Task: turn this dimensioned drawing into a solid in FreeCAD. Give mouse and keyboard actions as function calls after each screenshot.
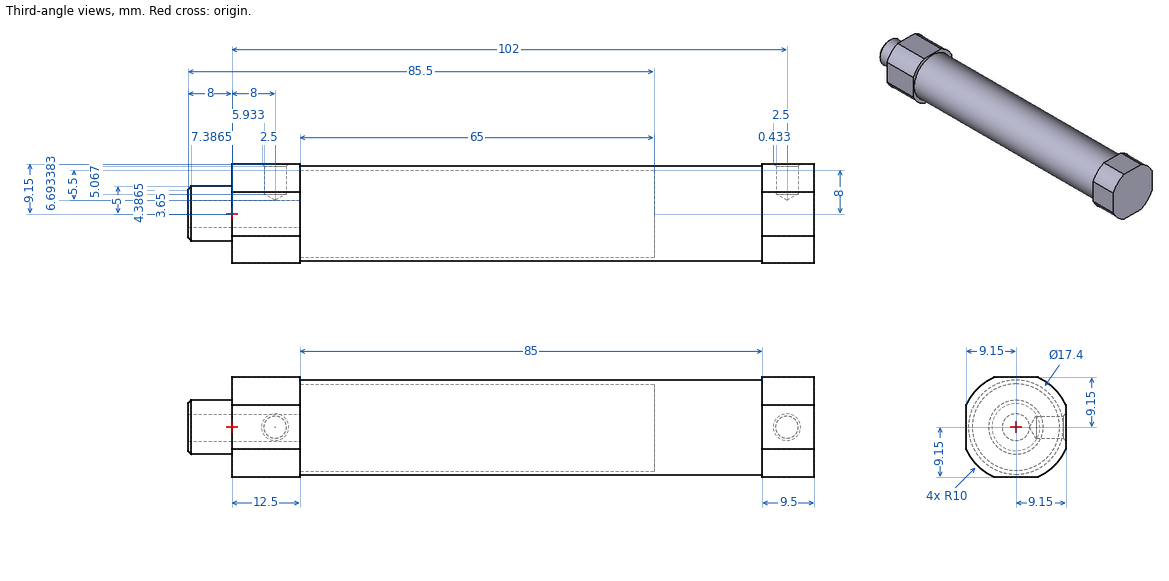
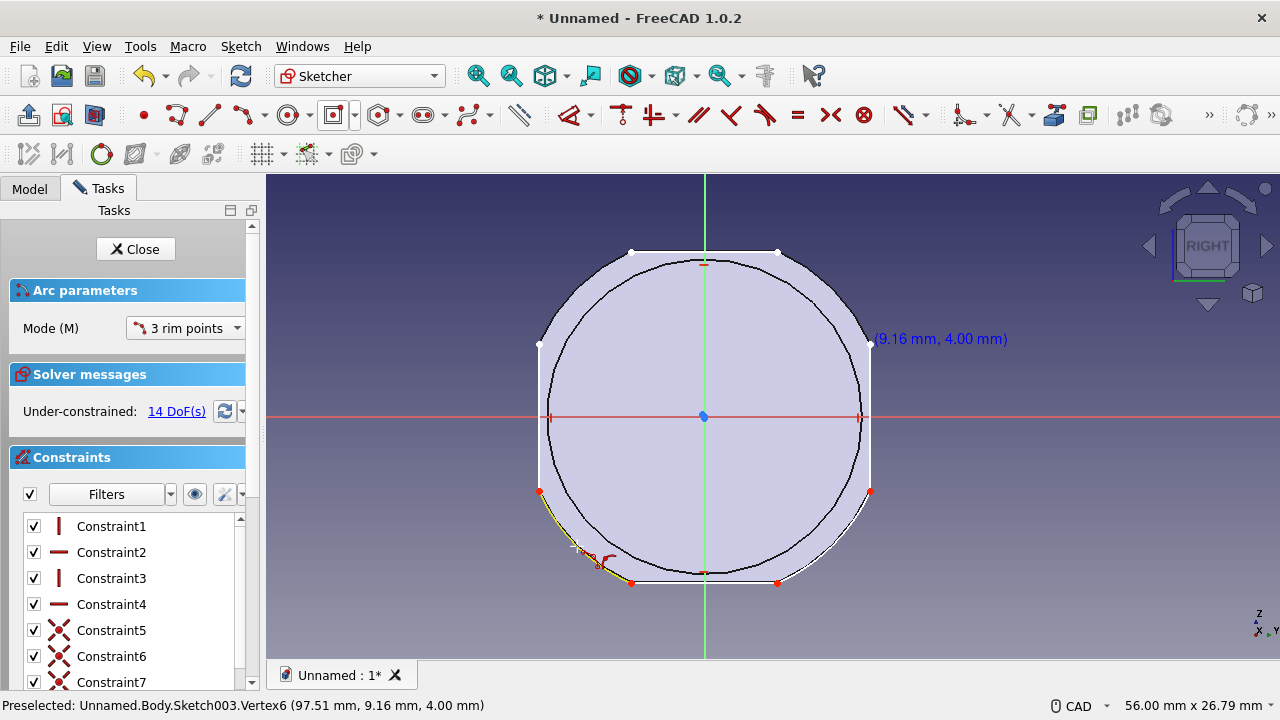
click(777, 252)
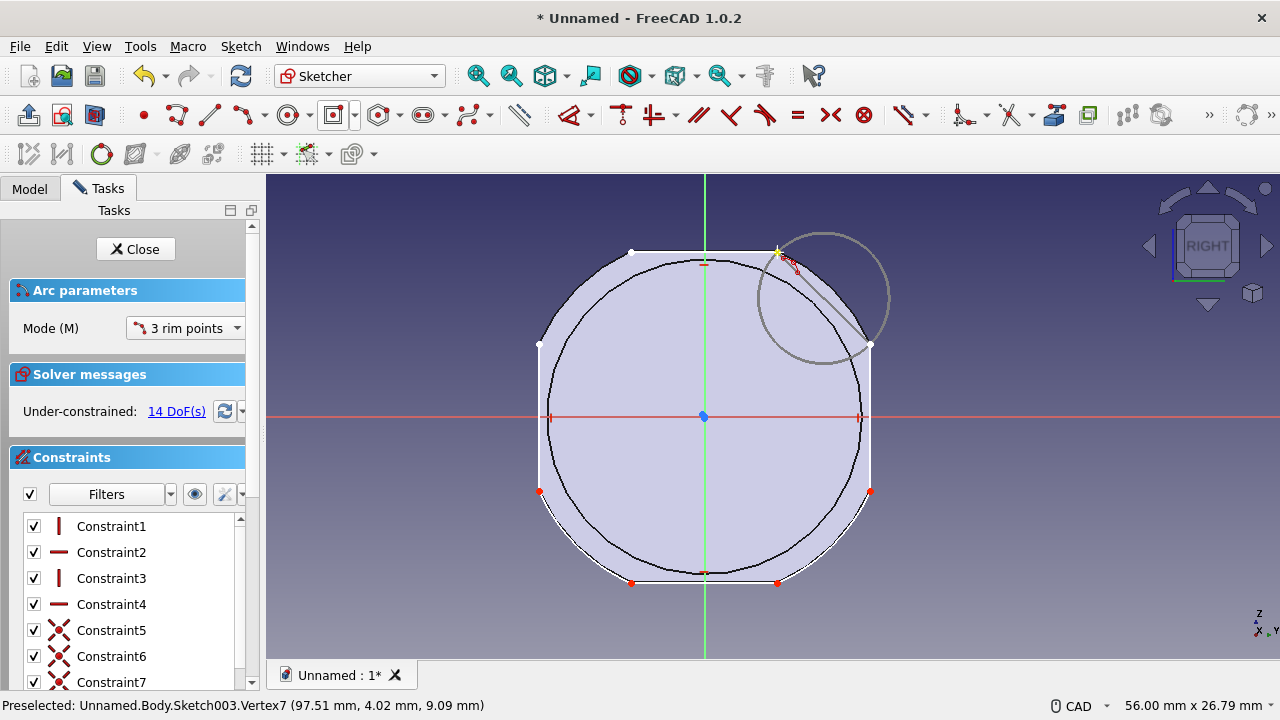
scroll(833, 289, up, 2)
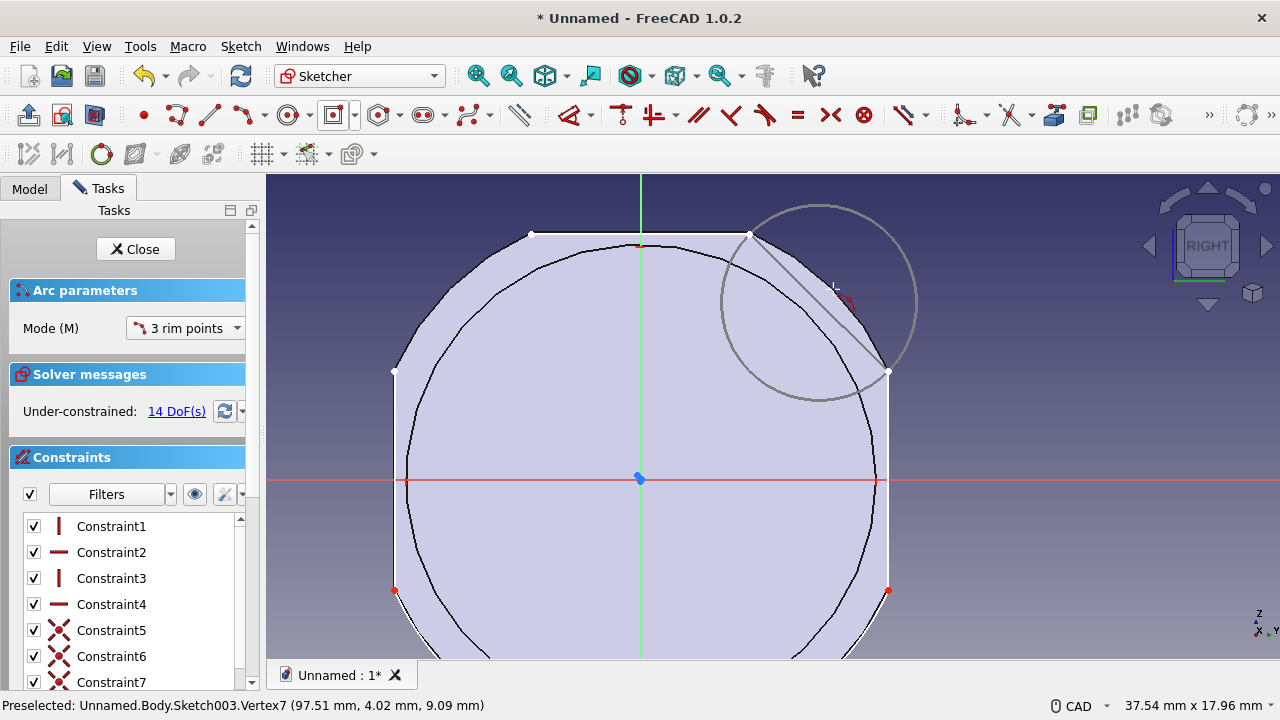
click(832, 289)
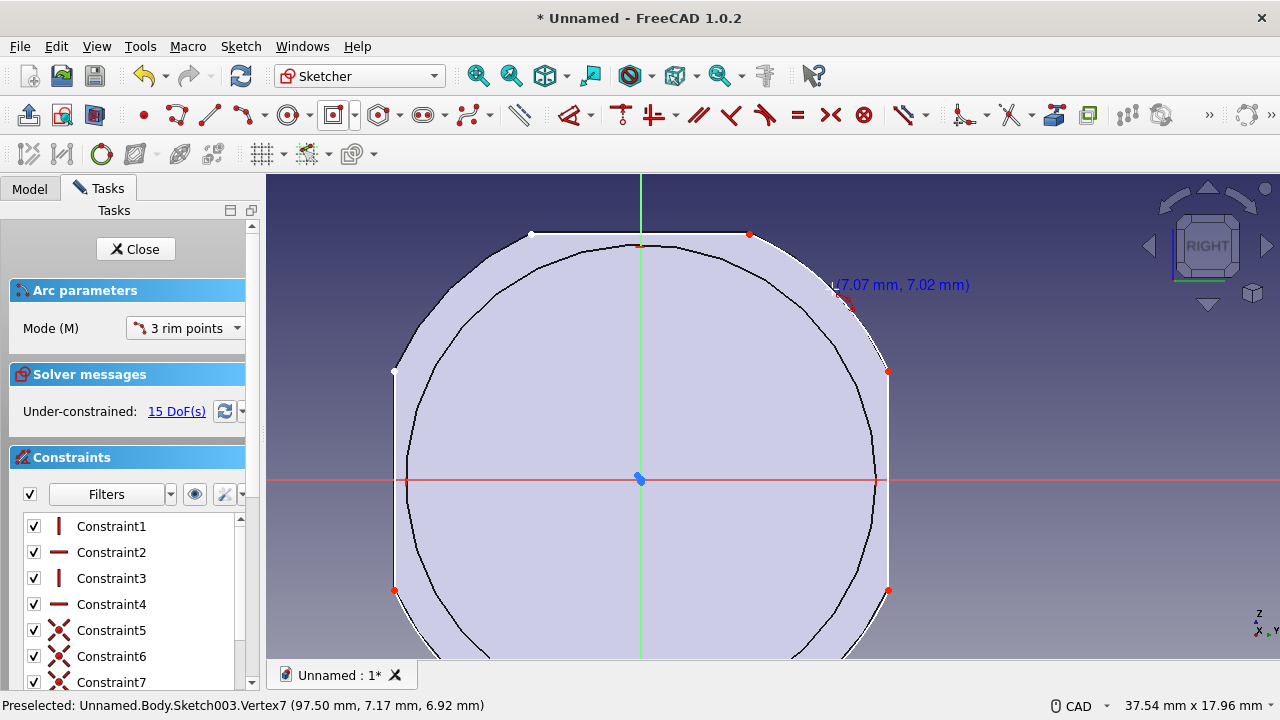
click(532, 234)
click(395, 371)
click(450, 289)
key(Escape)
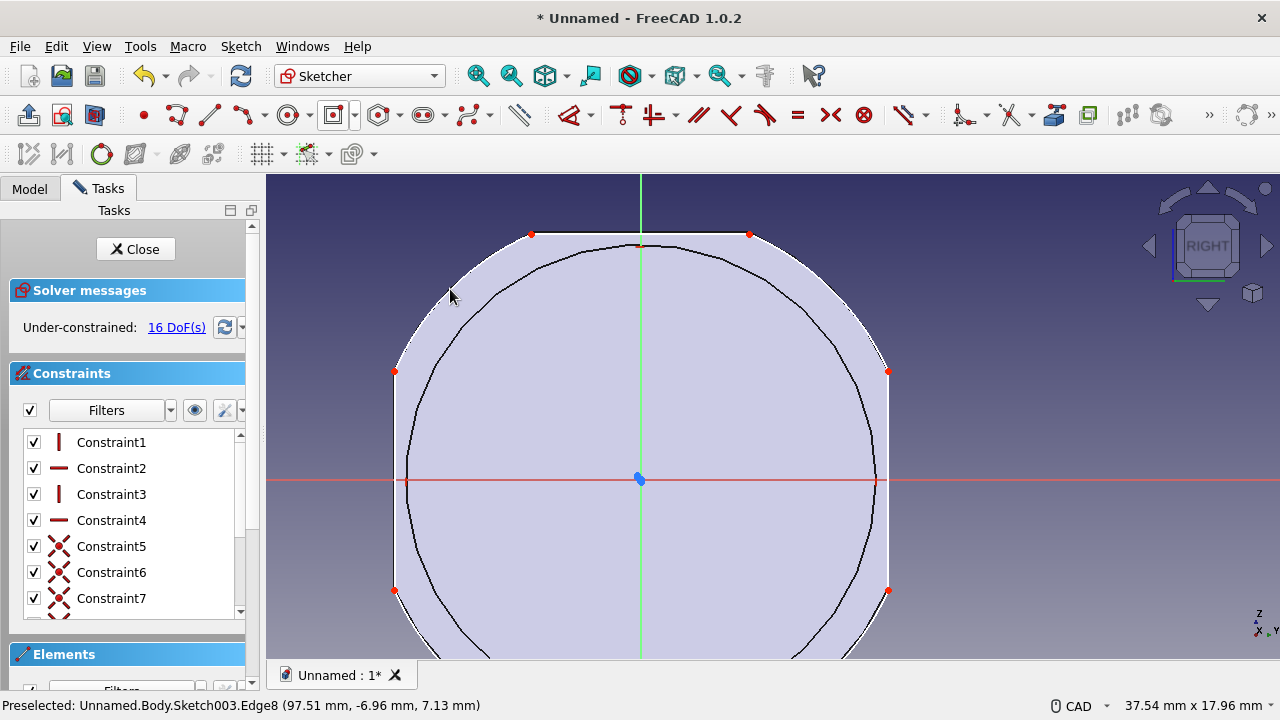
click(413, 626)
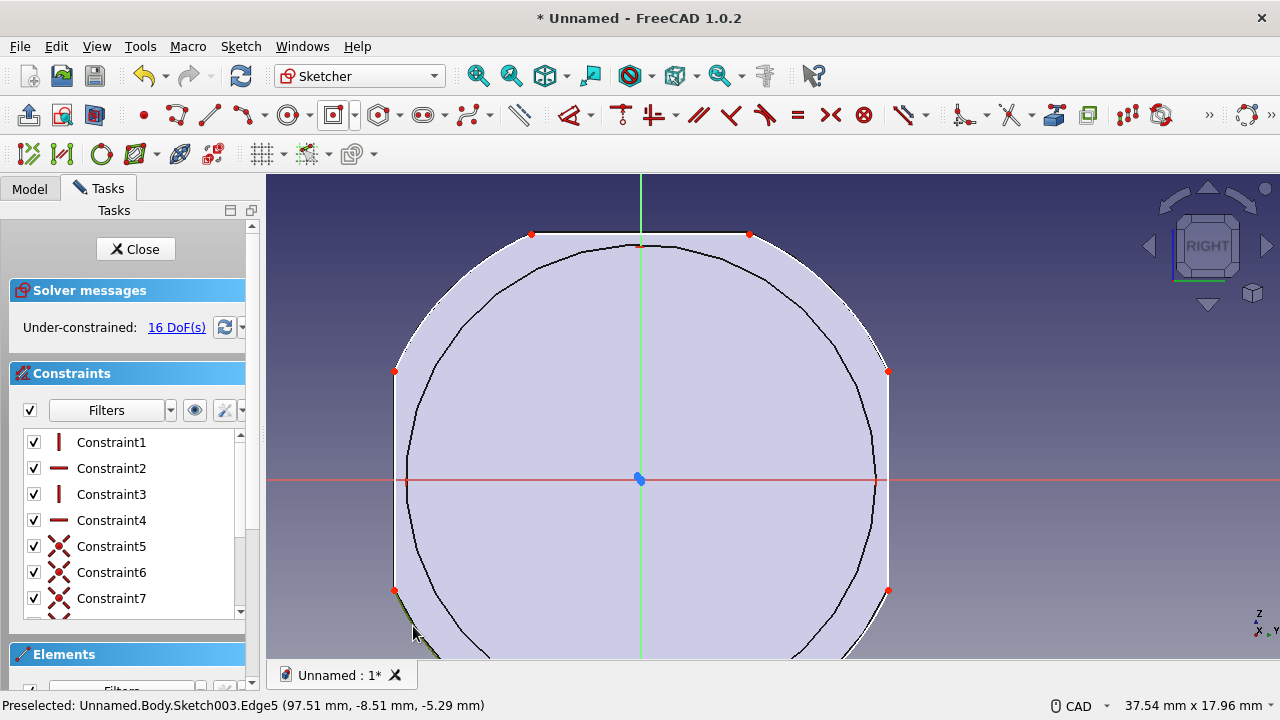
click(869, 626)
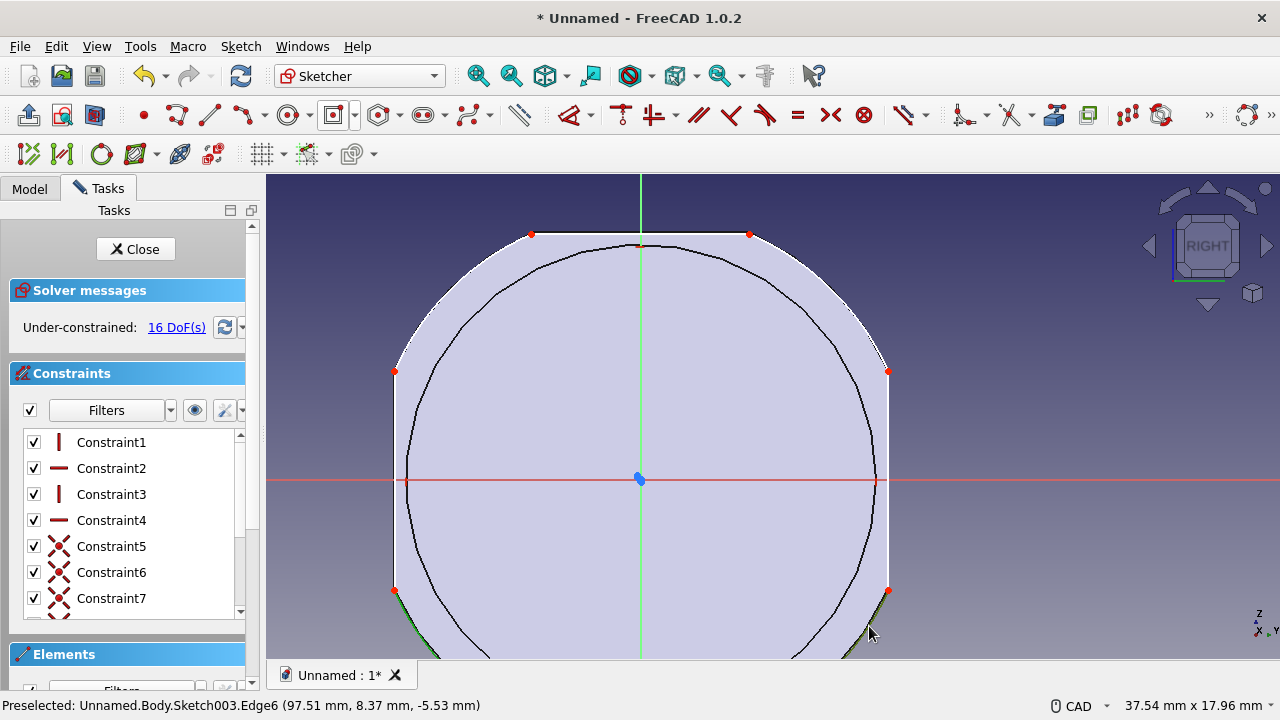
click(621, 116)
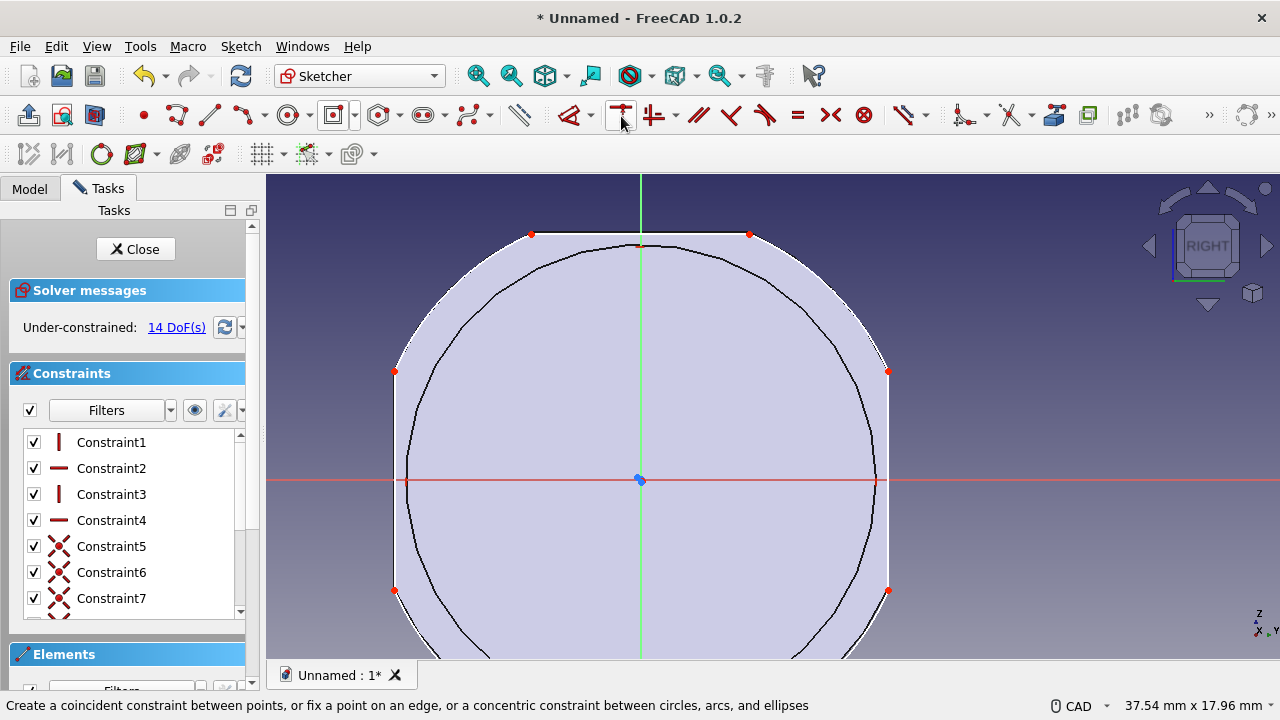
click(413, 626)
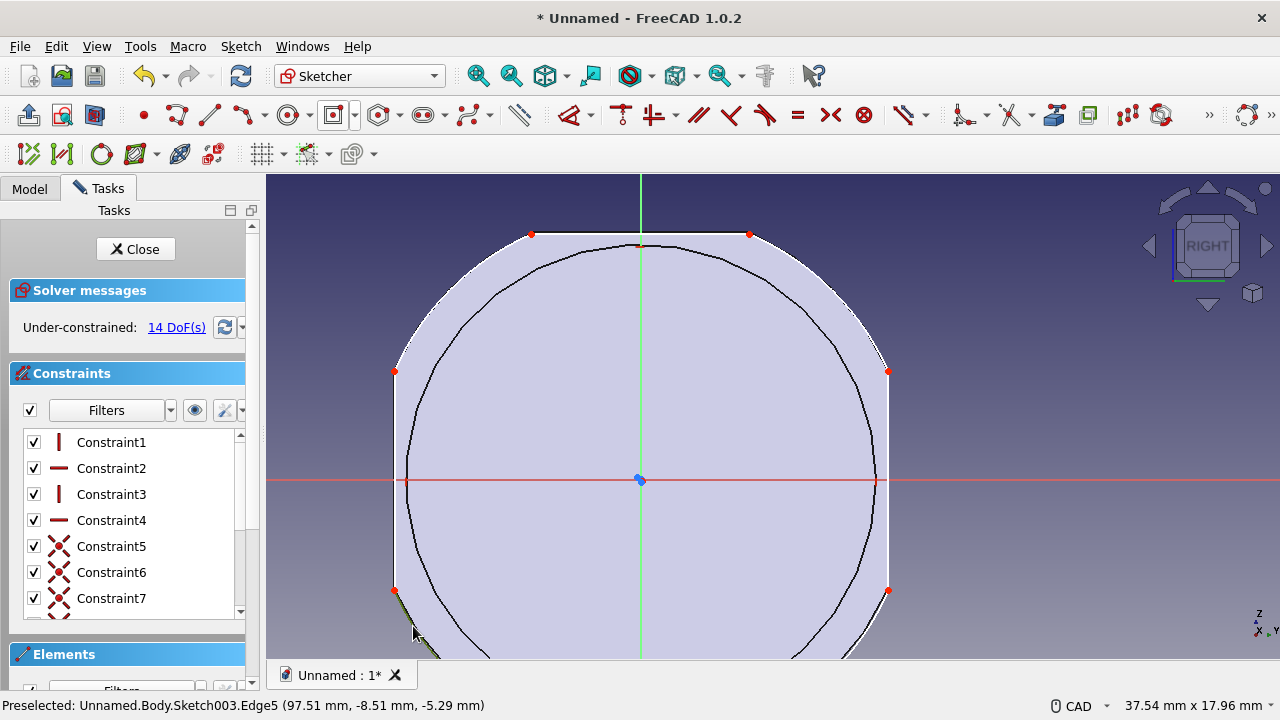
click(858, 320)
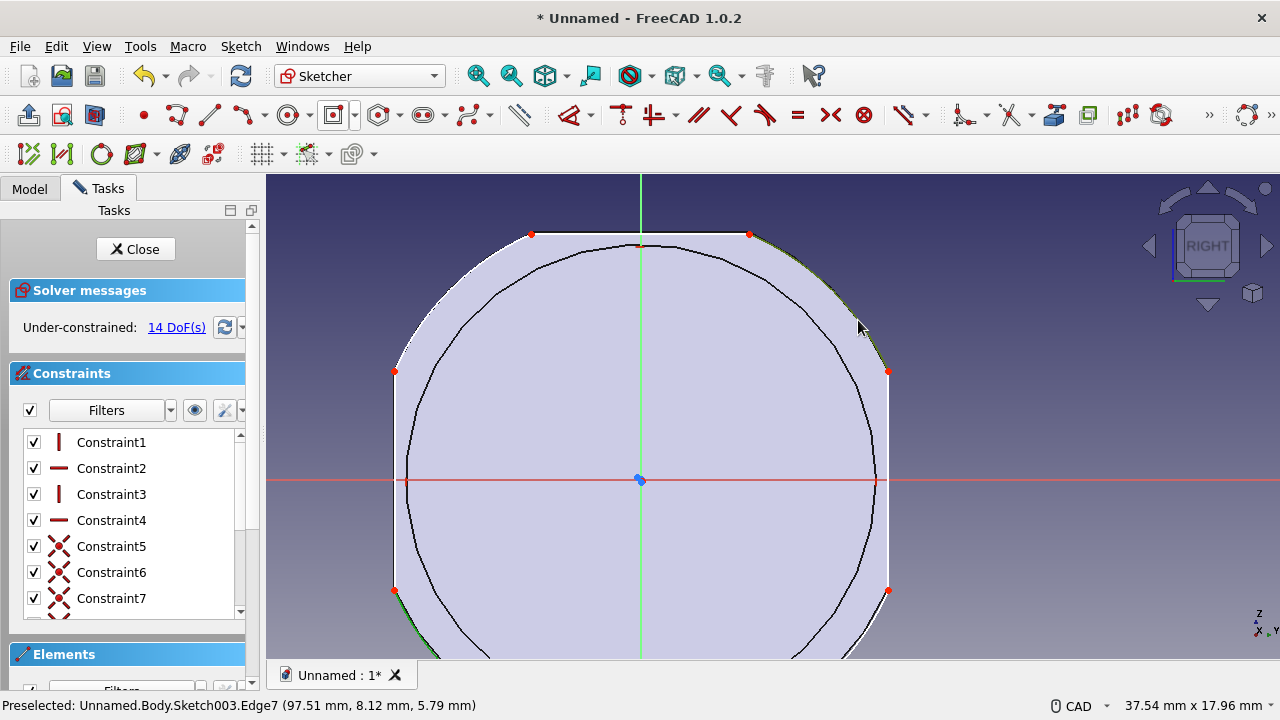
click(621, 116)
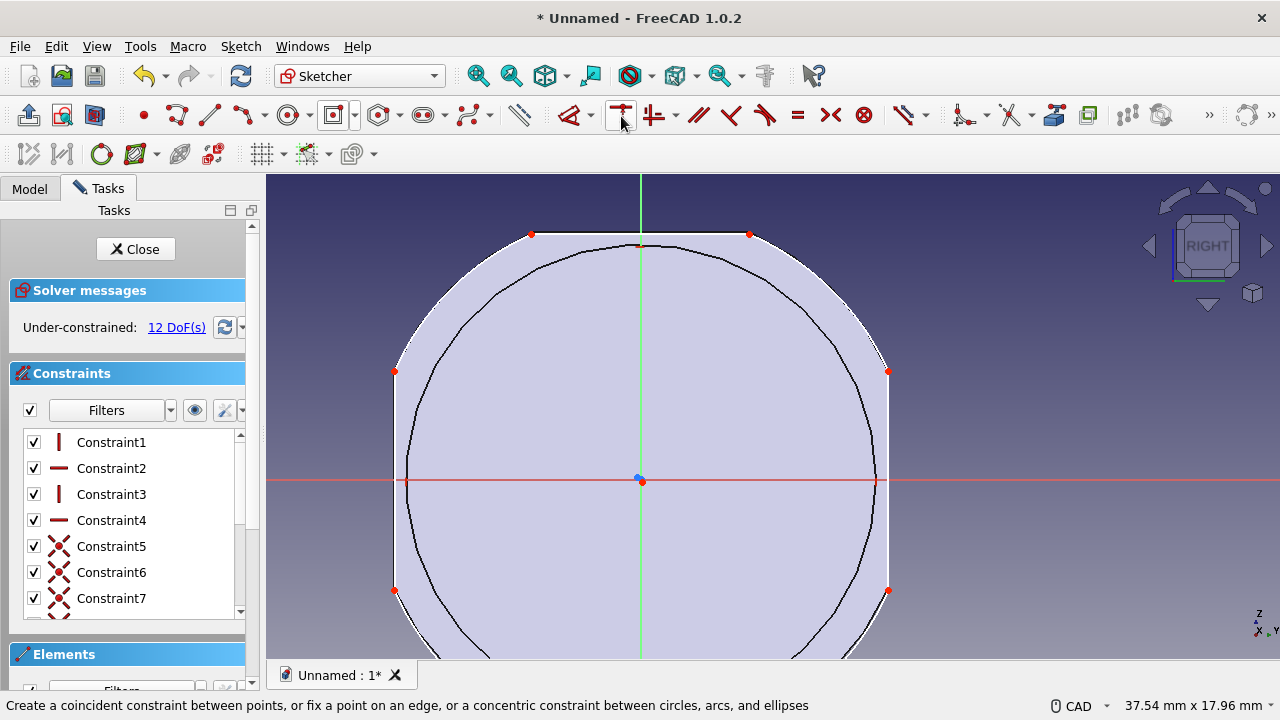
click(413, 626)